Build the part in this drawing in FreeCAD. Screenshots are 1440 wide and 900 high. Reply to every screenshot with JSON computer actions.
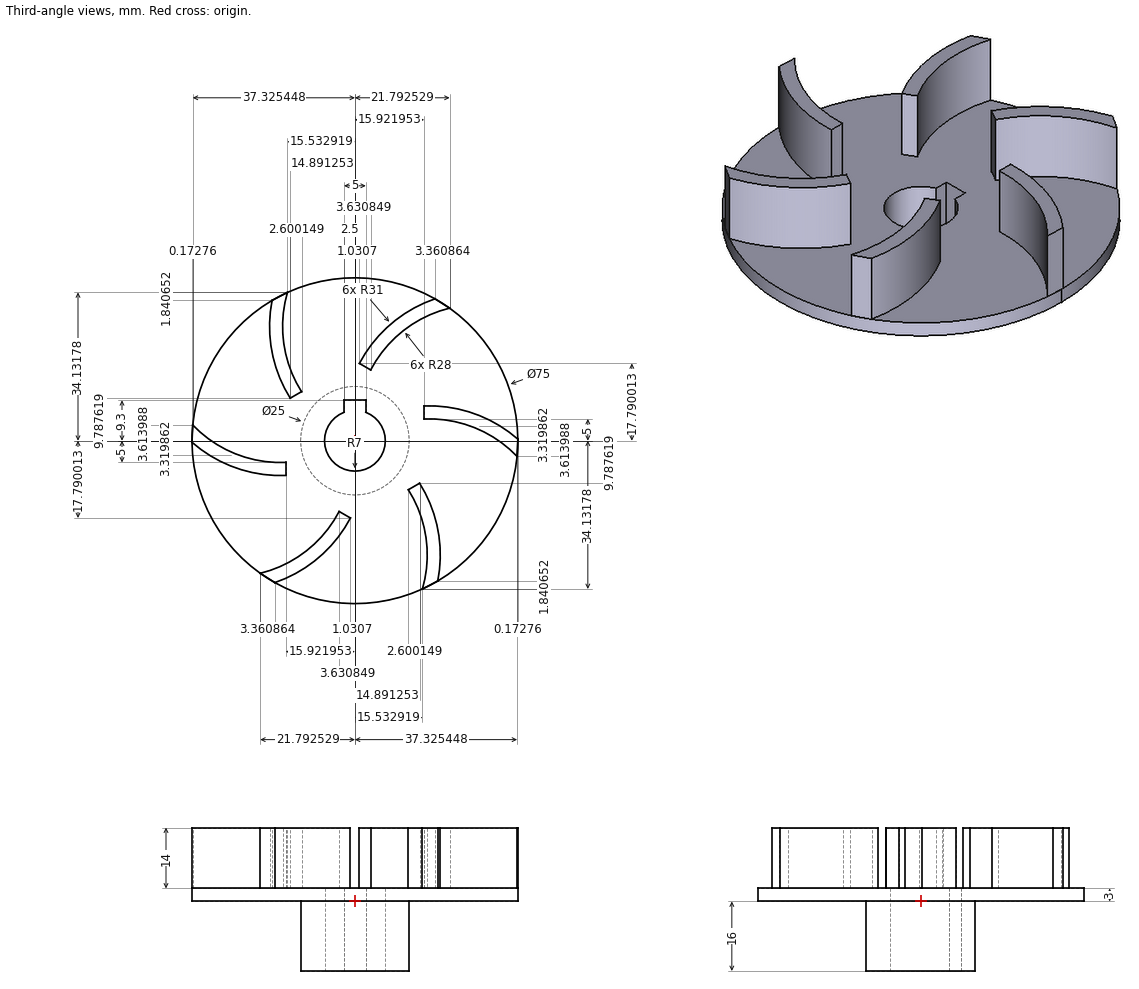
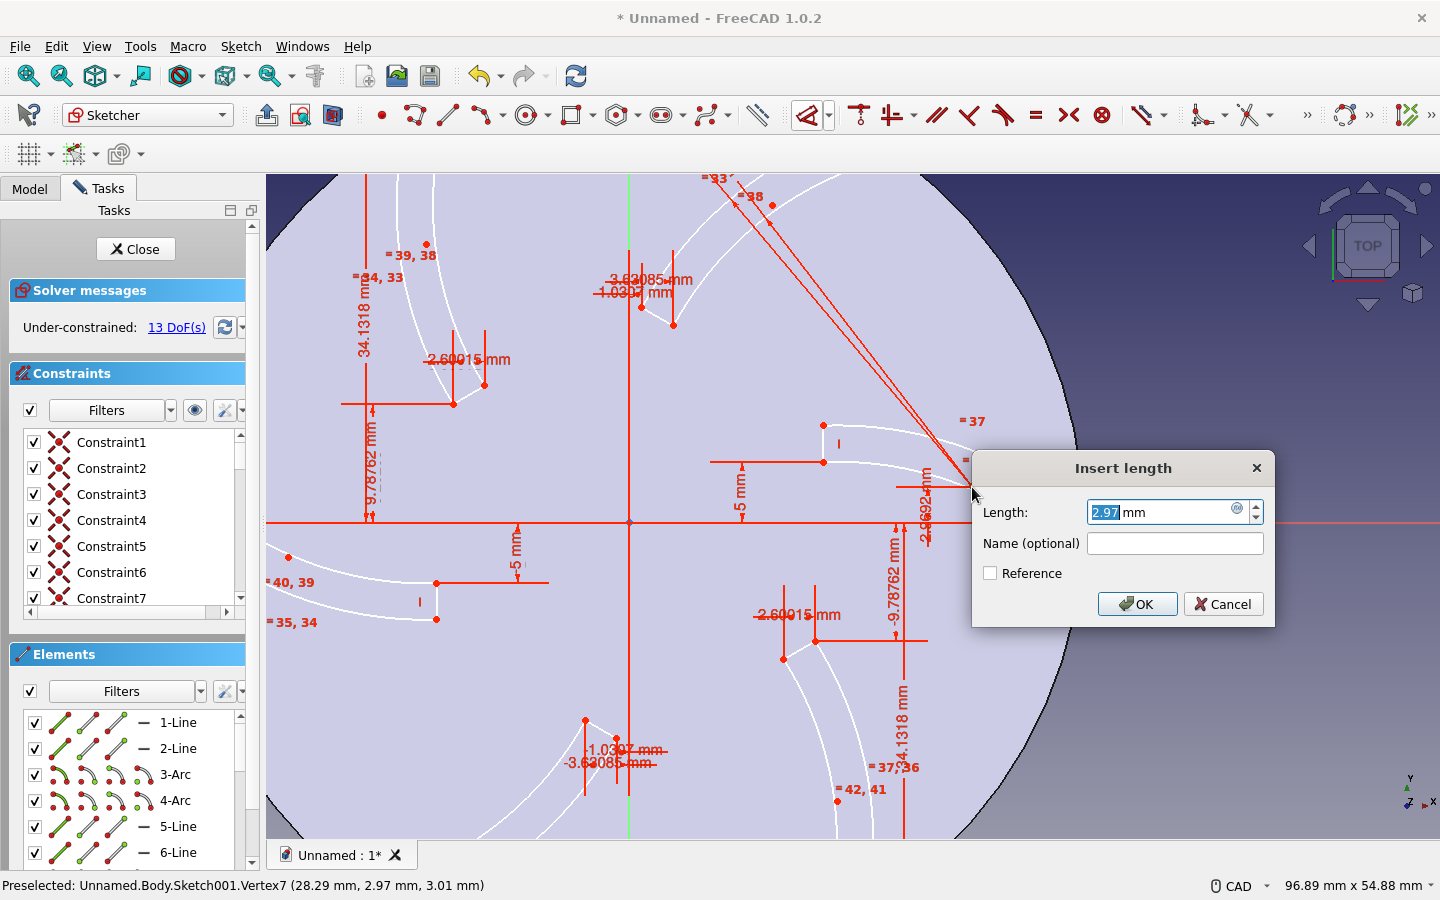
{"action": "type", "text": "3.319862"}
{"action": "key", "text": "Return"}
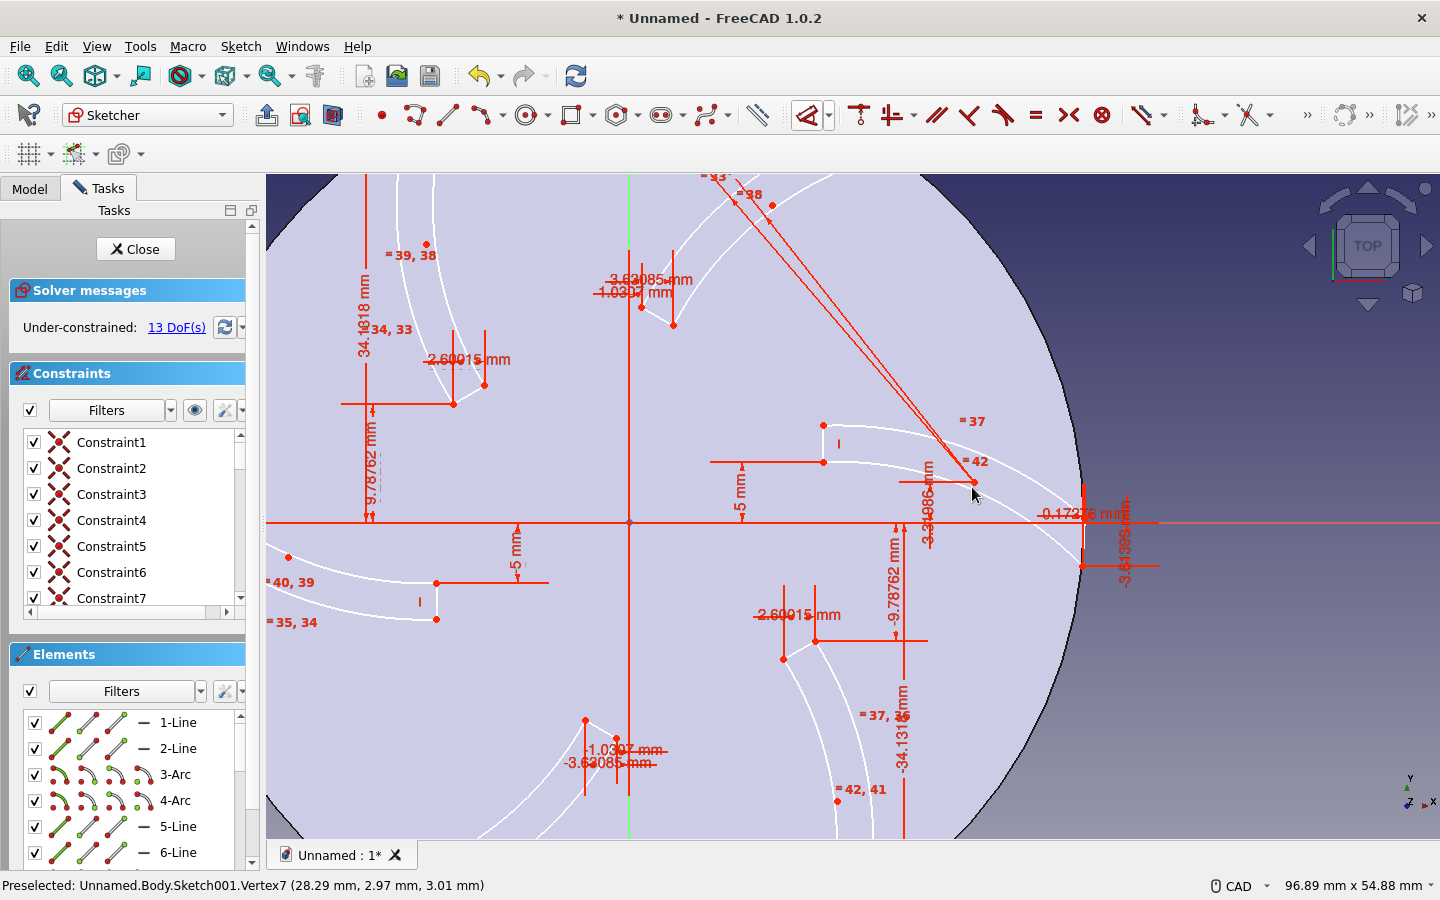
{"action": "scroll", "coordinate": [973, 487], "scroll_direction": "down", "scroll_amount": 3}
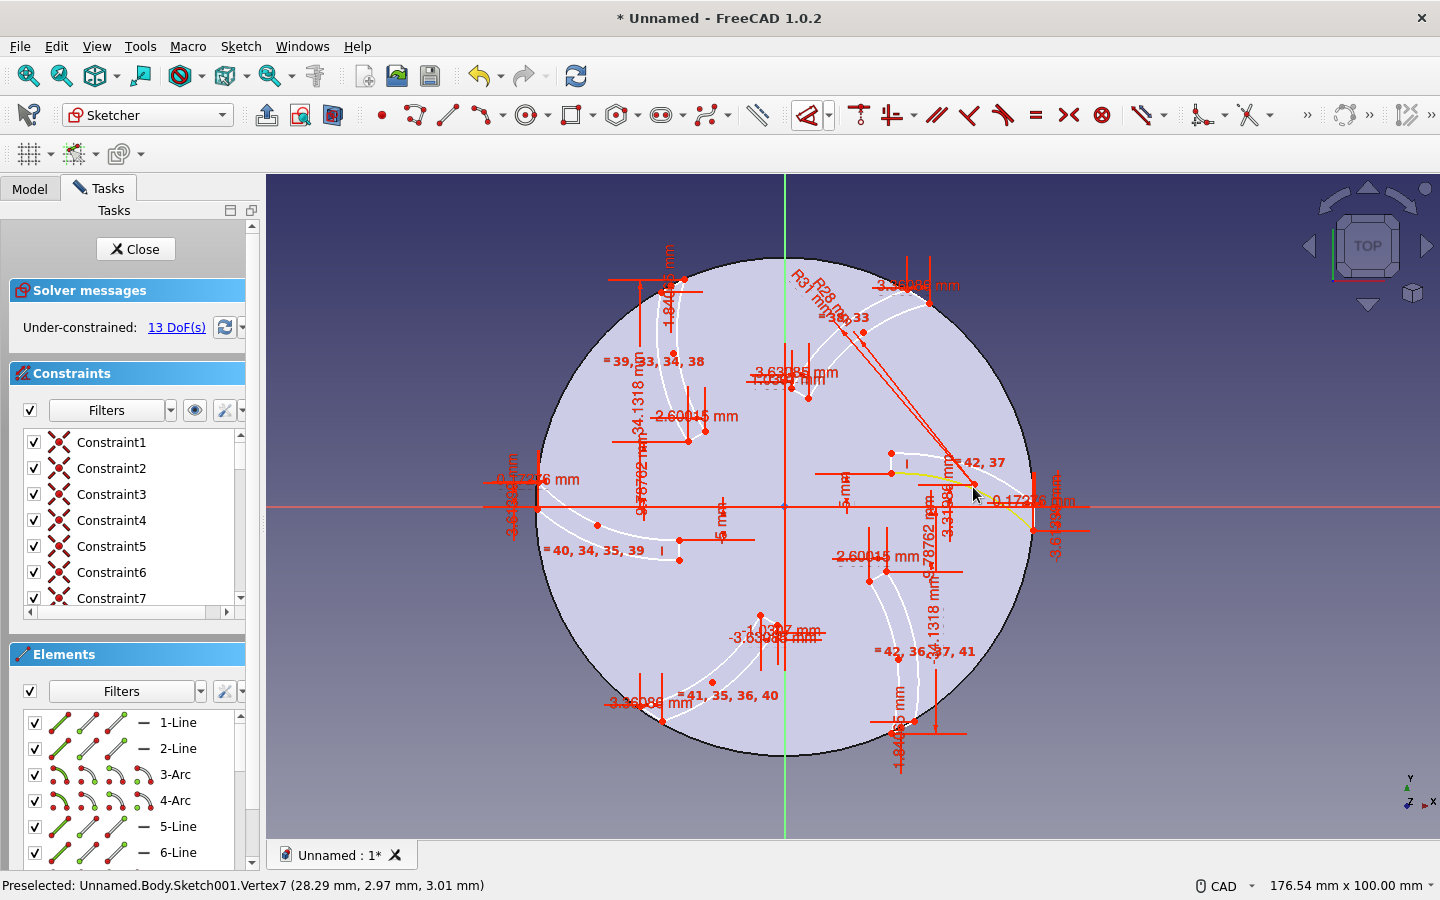
{"action": "scroll", "coordinate": [597, 526], "scroll_direction": "up", "scroll_amount": 3}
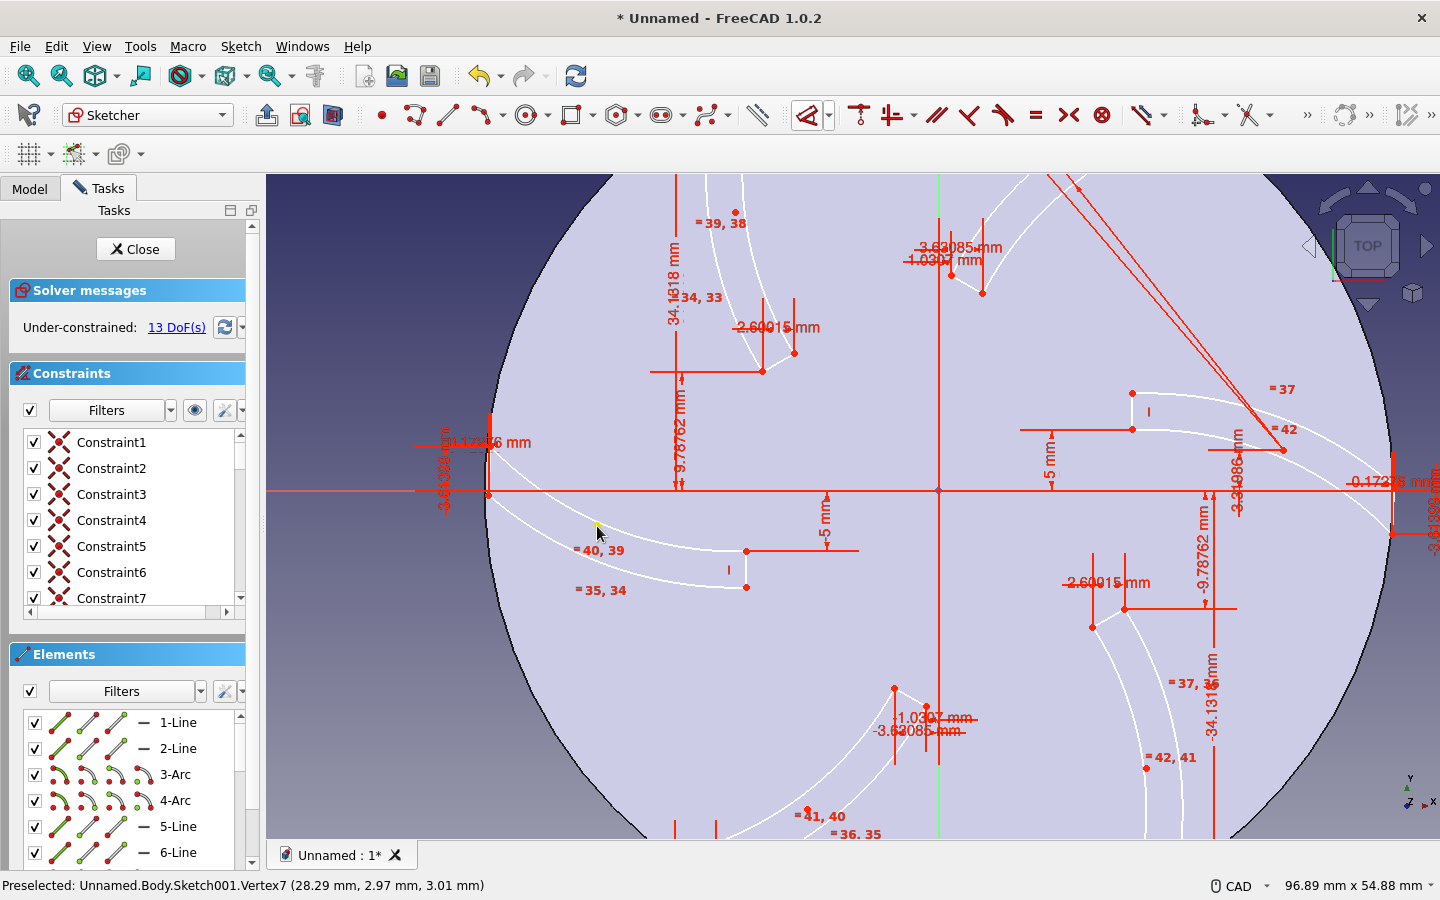
{"action": "left_click", "coordinate": [597, 525]}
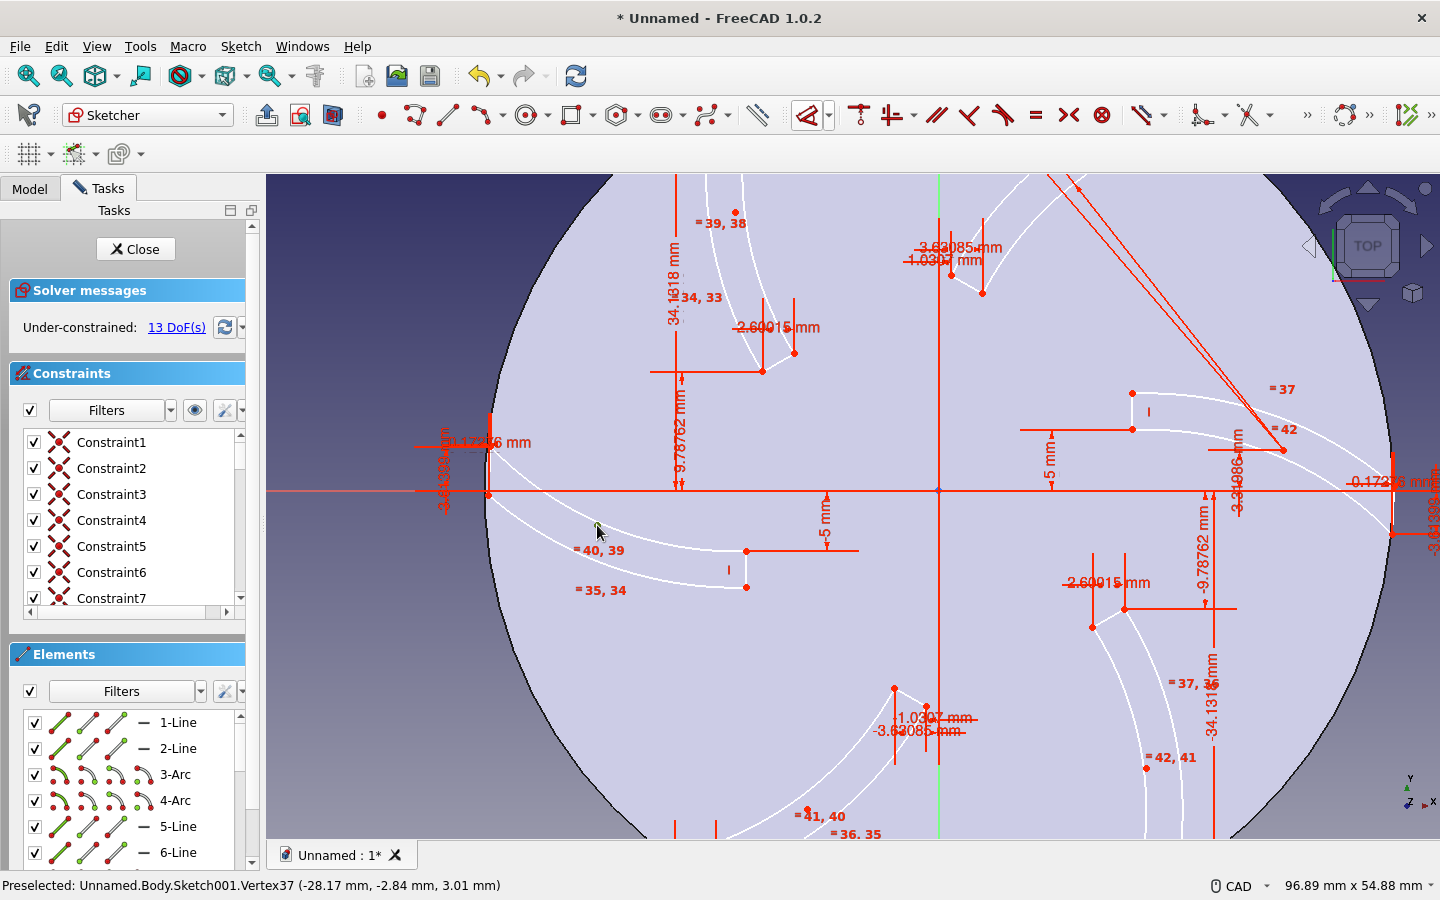
{"action": "key", "text": "i"}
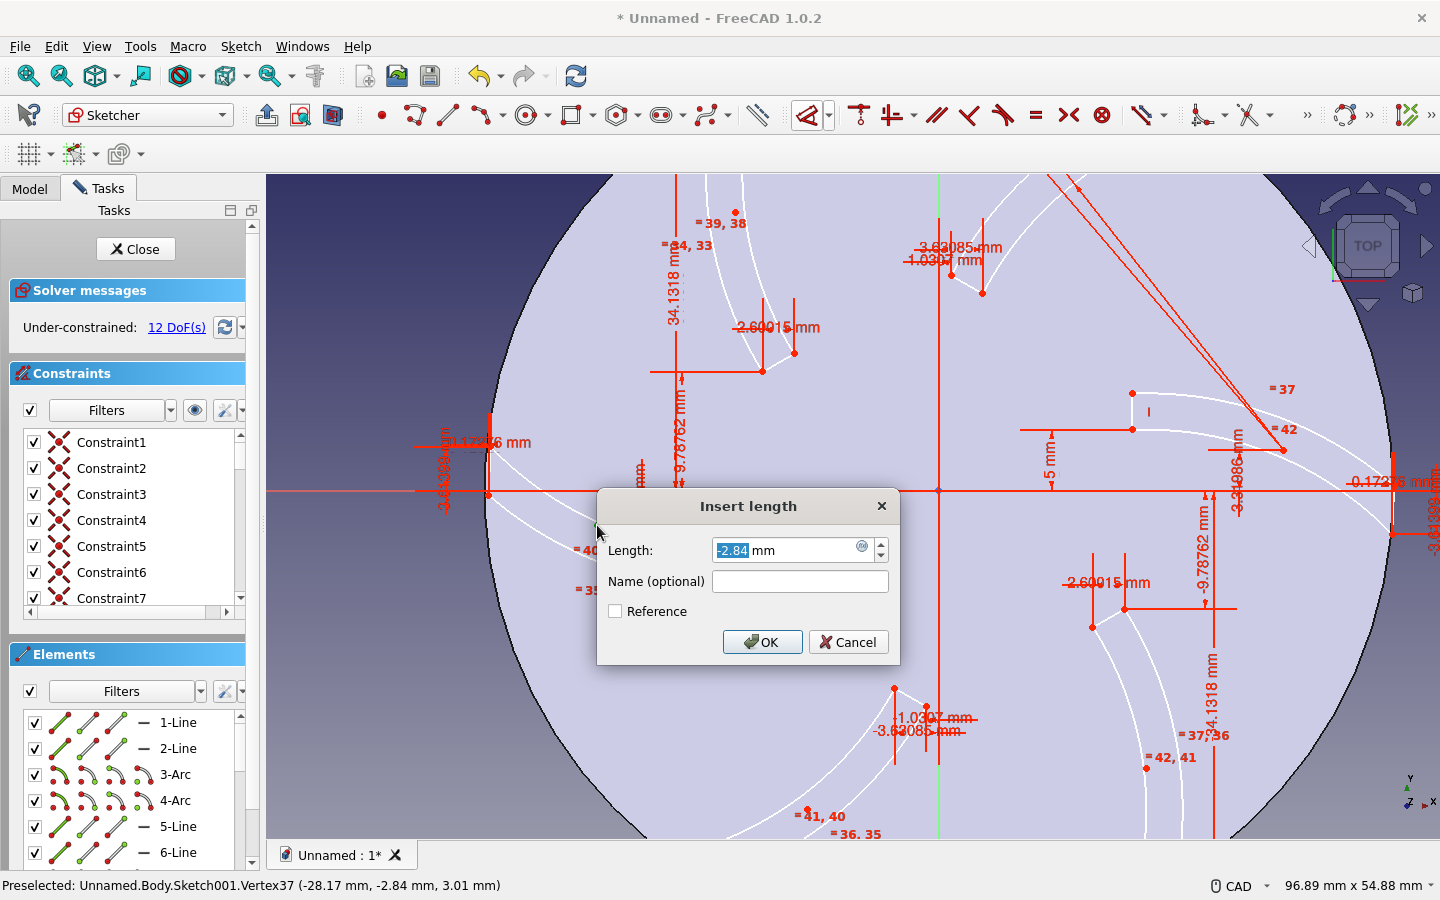
{"action": "type", "text": "-3.319862"}
{"action": "key", "text": "Return"}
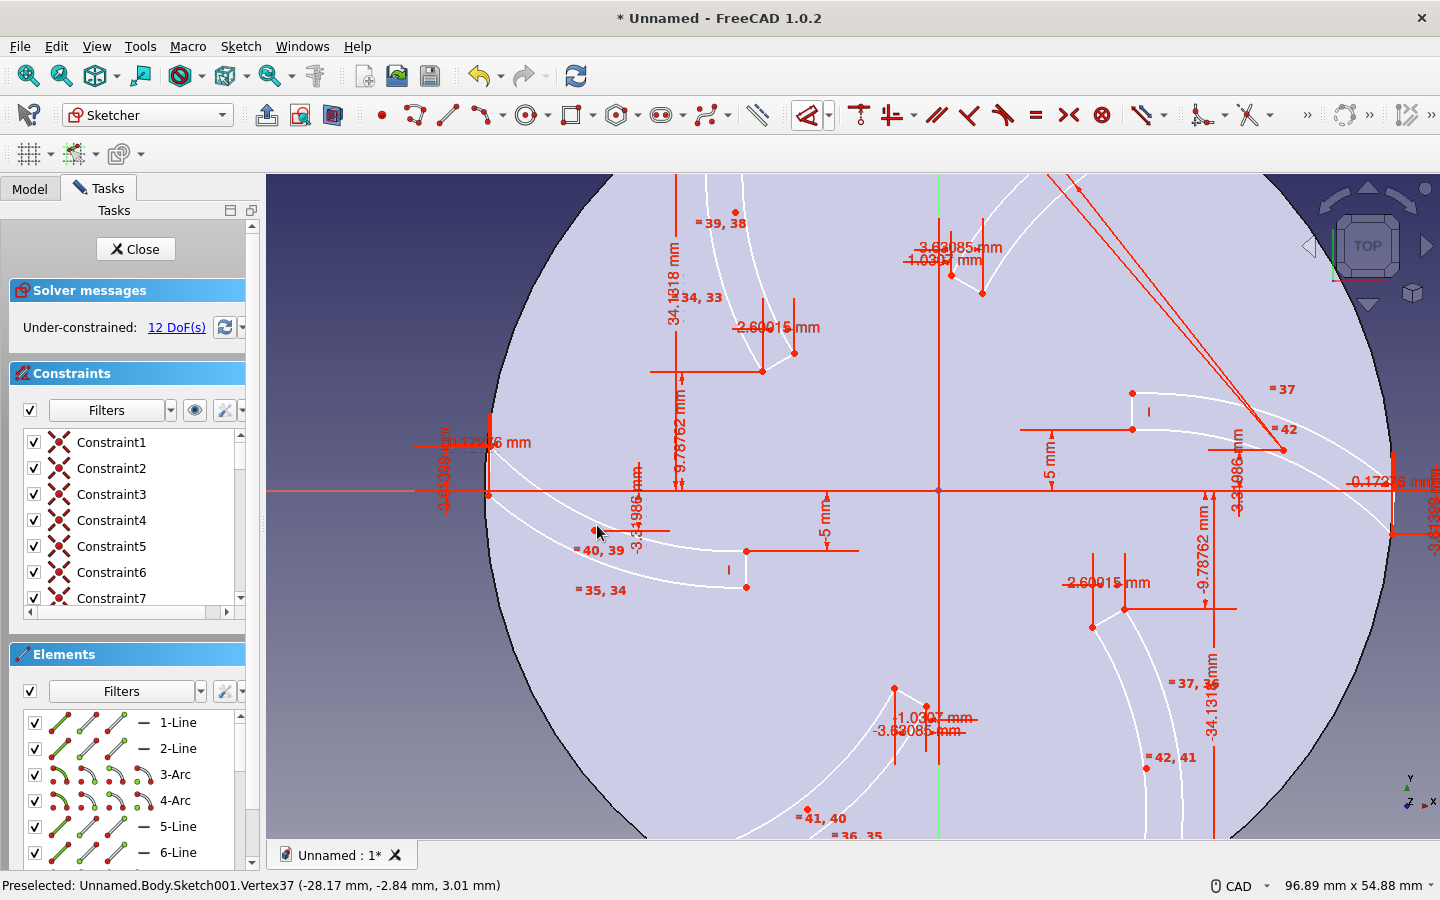
{"action": "scroll", "coordinate": [597, 526], "scroll_direction": "down", "scroll_amount": 3}